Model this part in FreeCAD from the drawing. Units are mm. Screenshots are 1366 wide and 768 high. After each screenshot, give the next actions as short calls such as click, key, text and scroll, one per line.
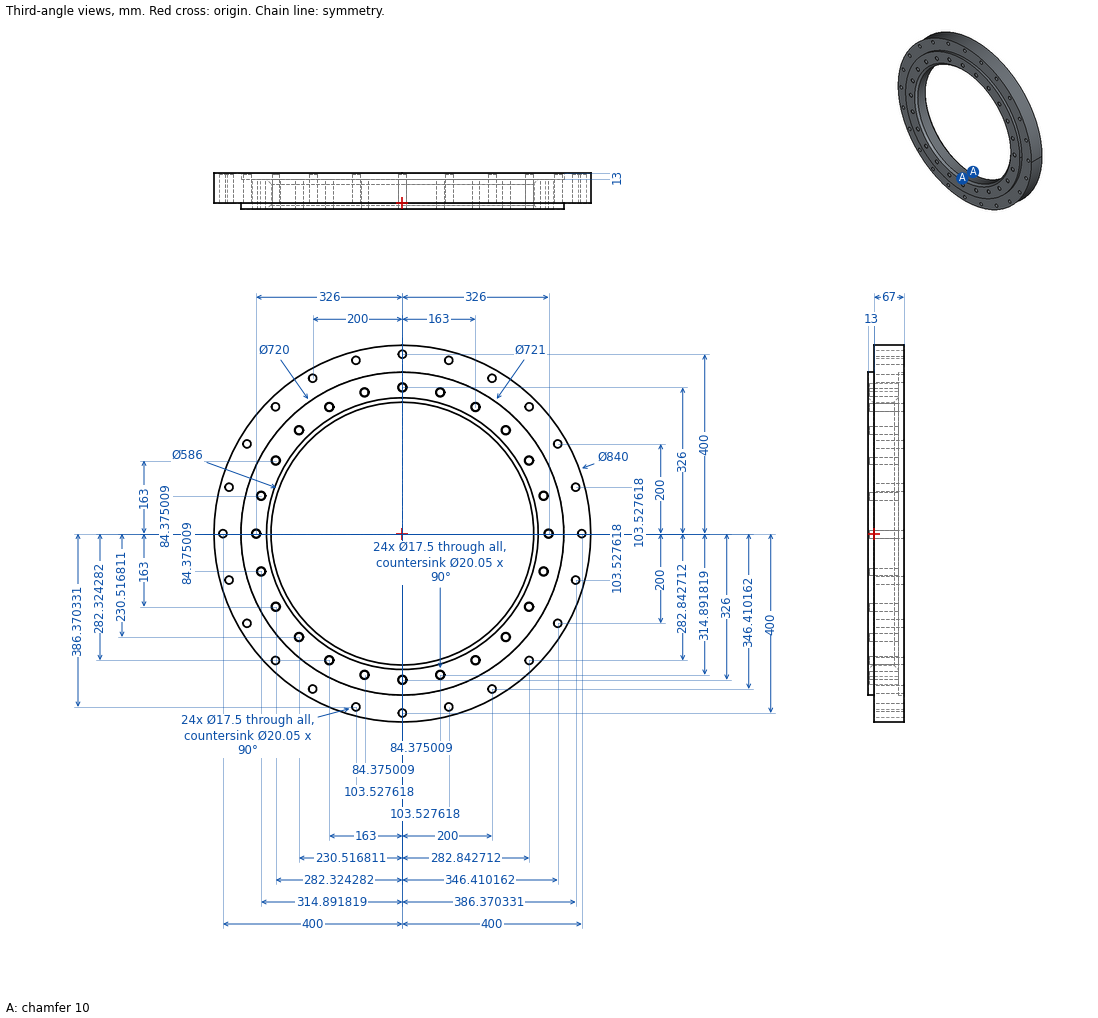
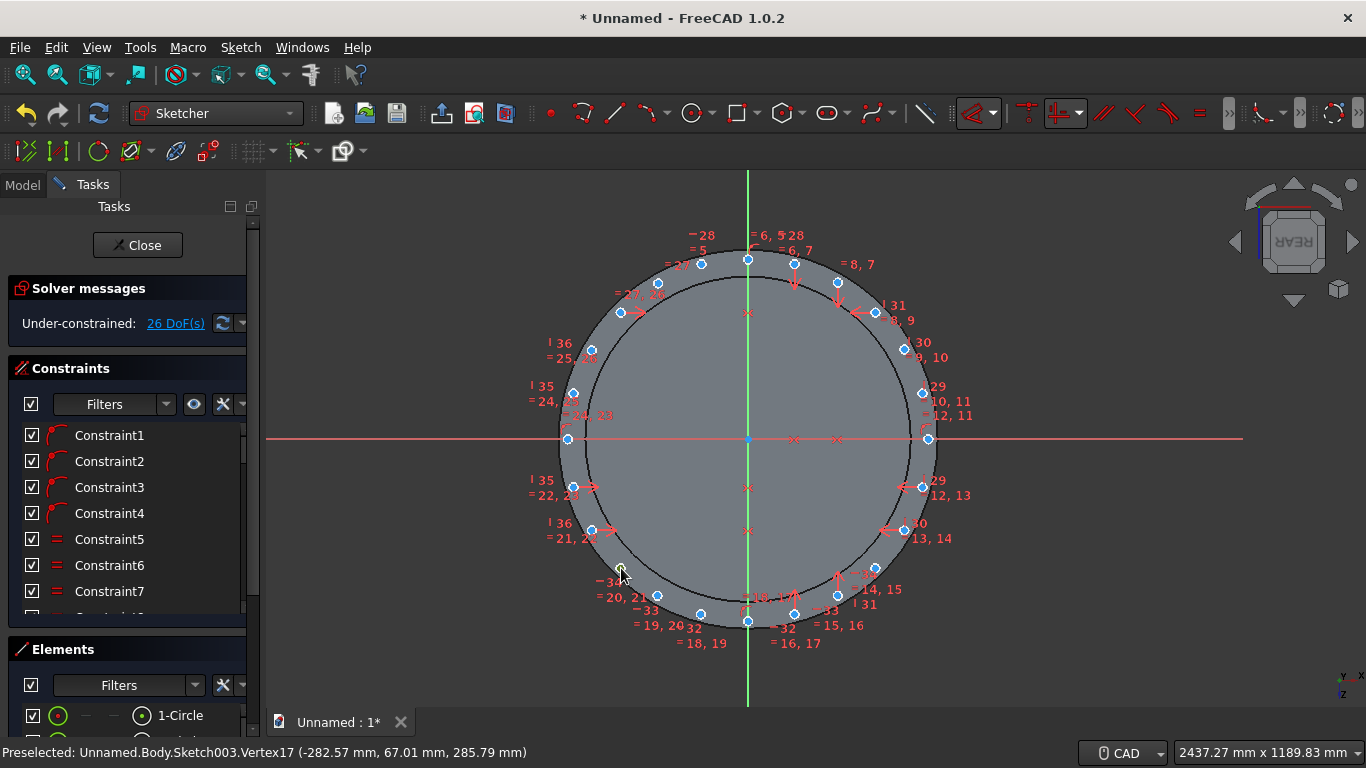
click(621, 313)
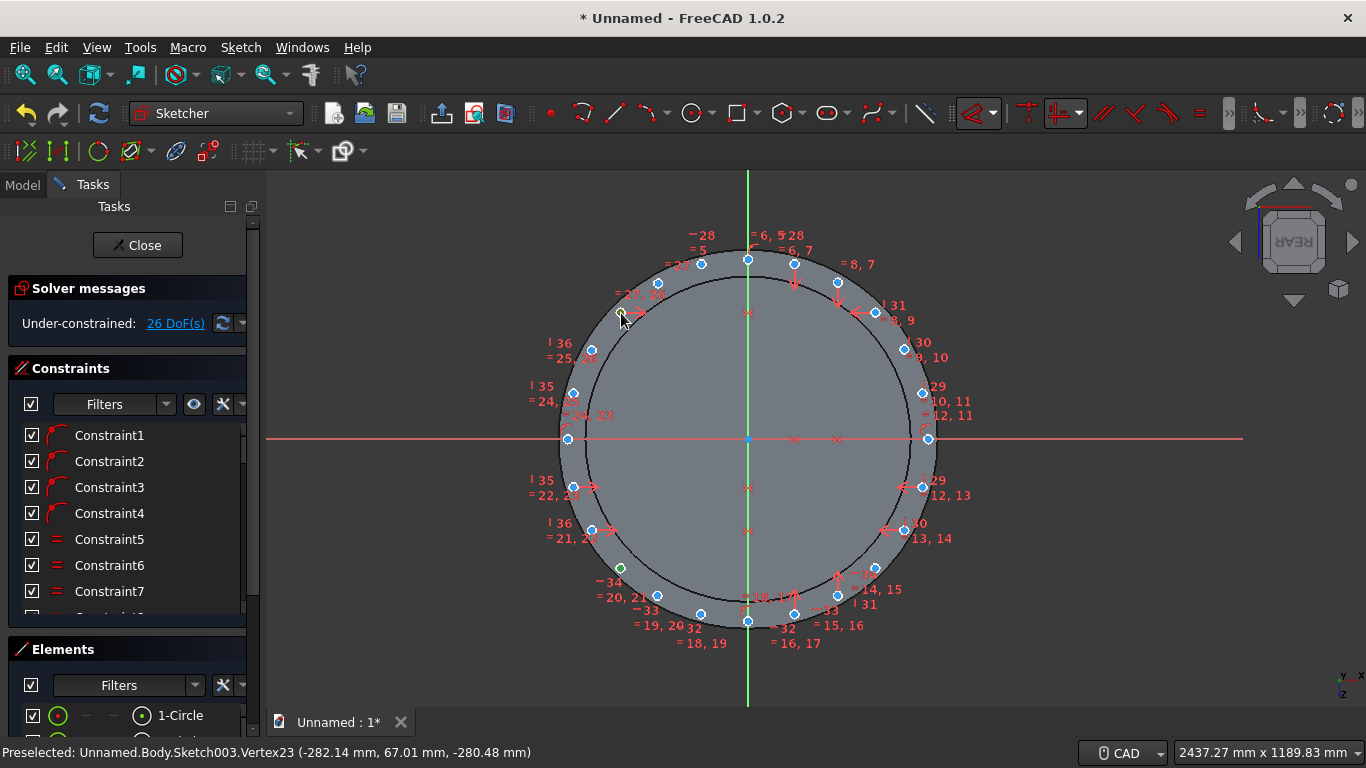
click(359, 439)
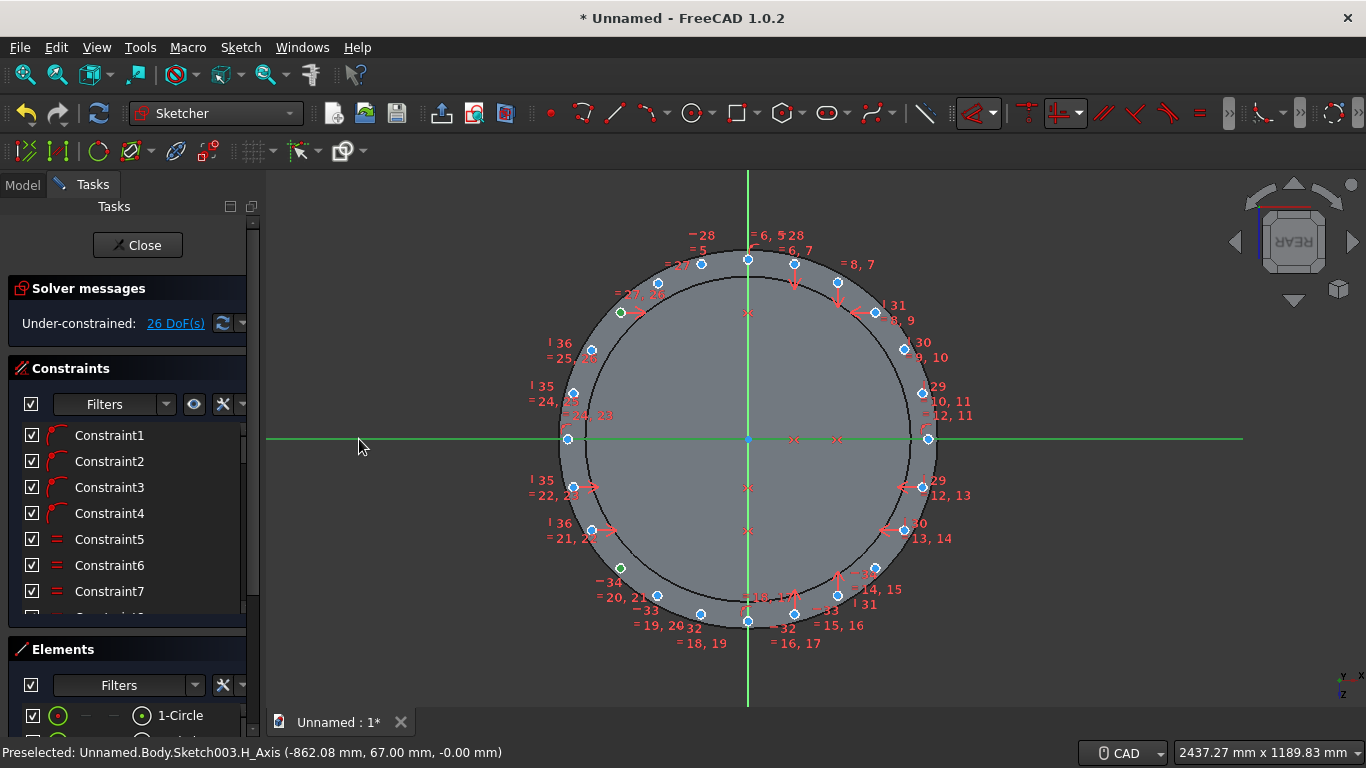
key(s)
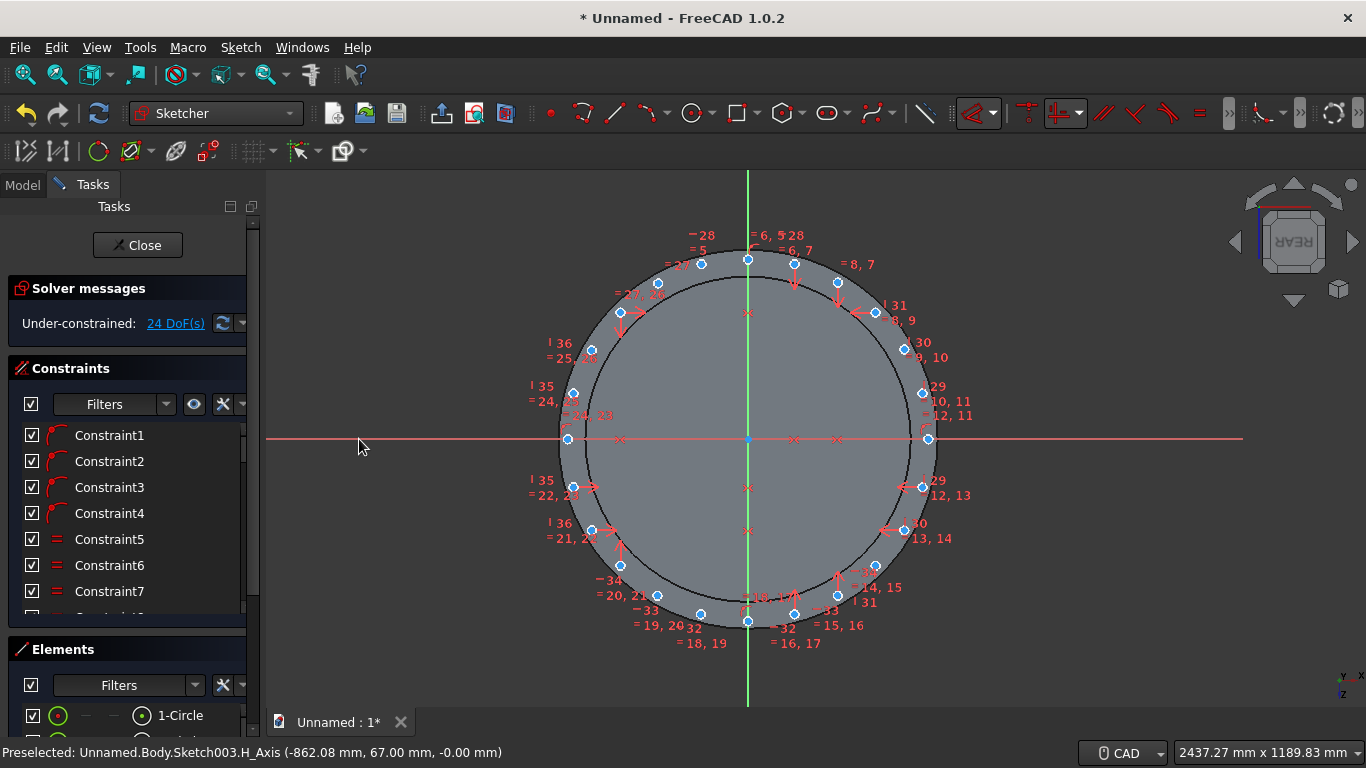
click(838, 283)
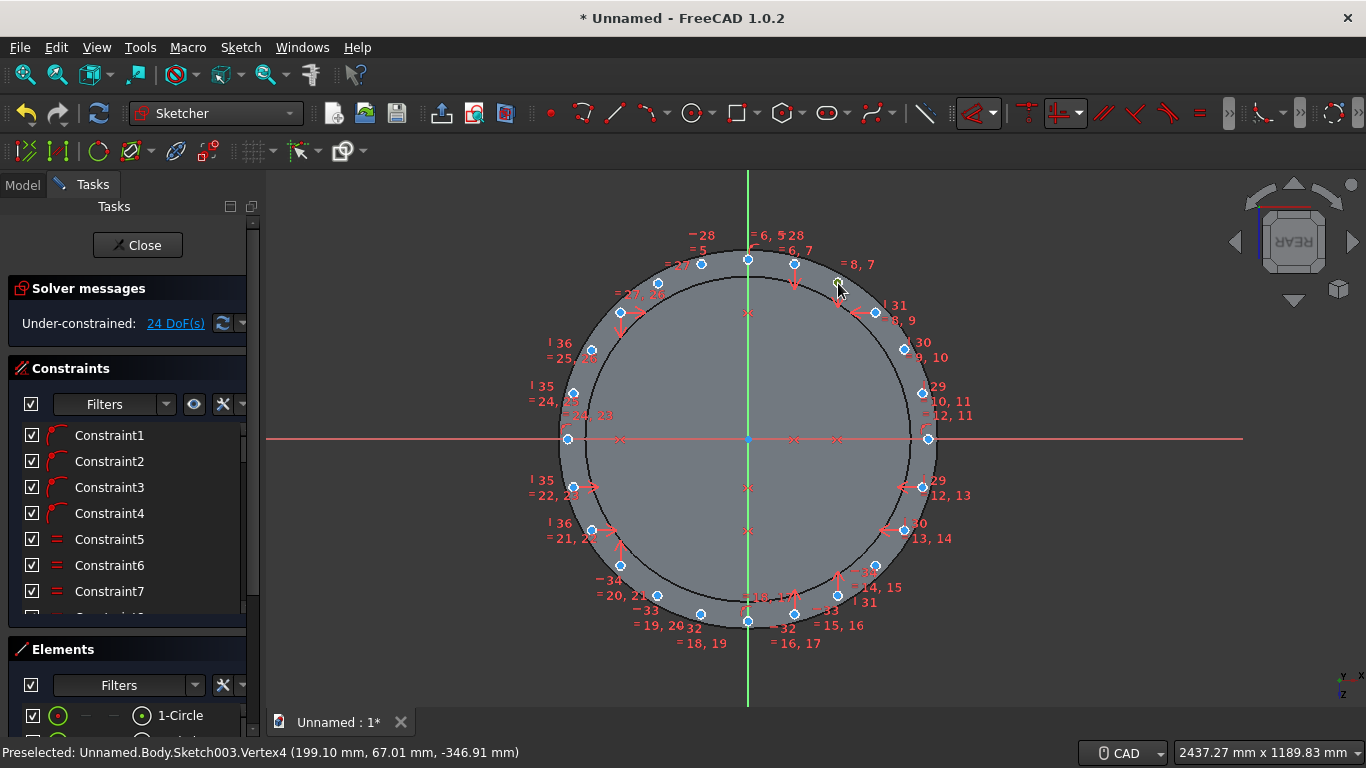
click(658, 283)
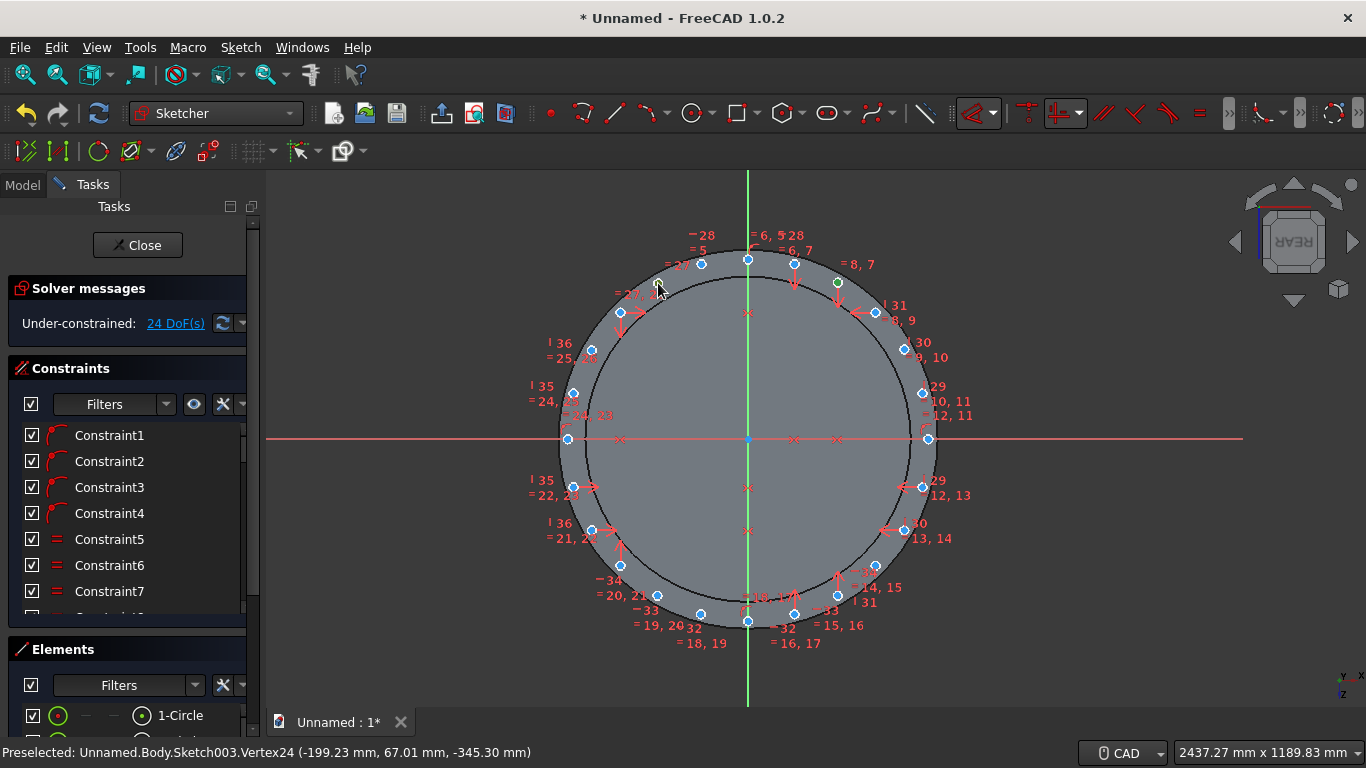
click(748, 576)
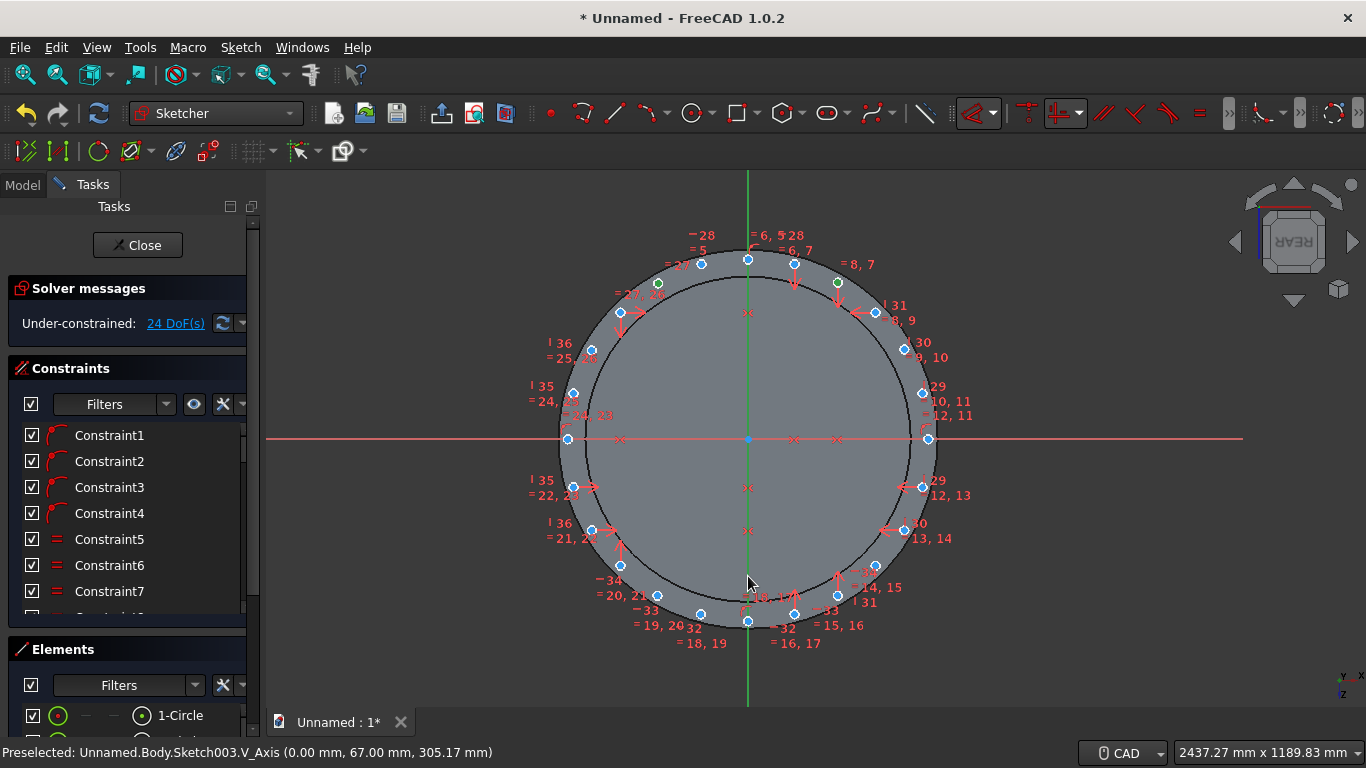
key(s)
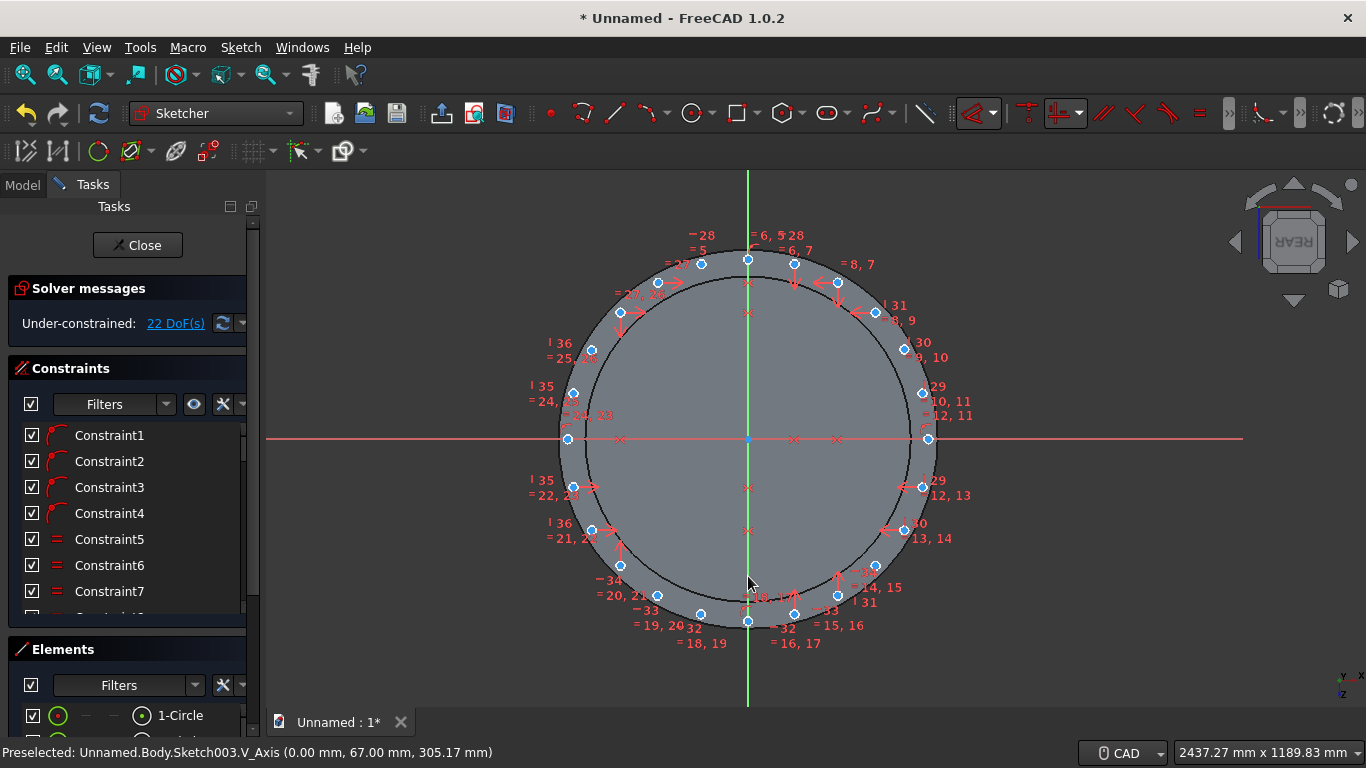
scroll(705, 261, up, 9)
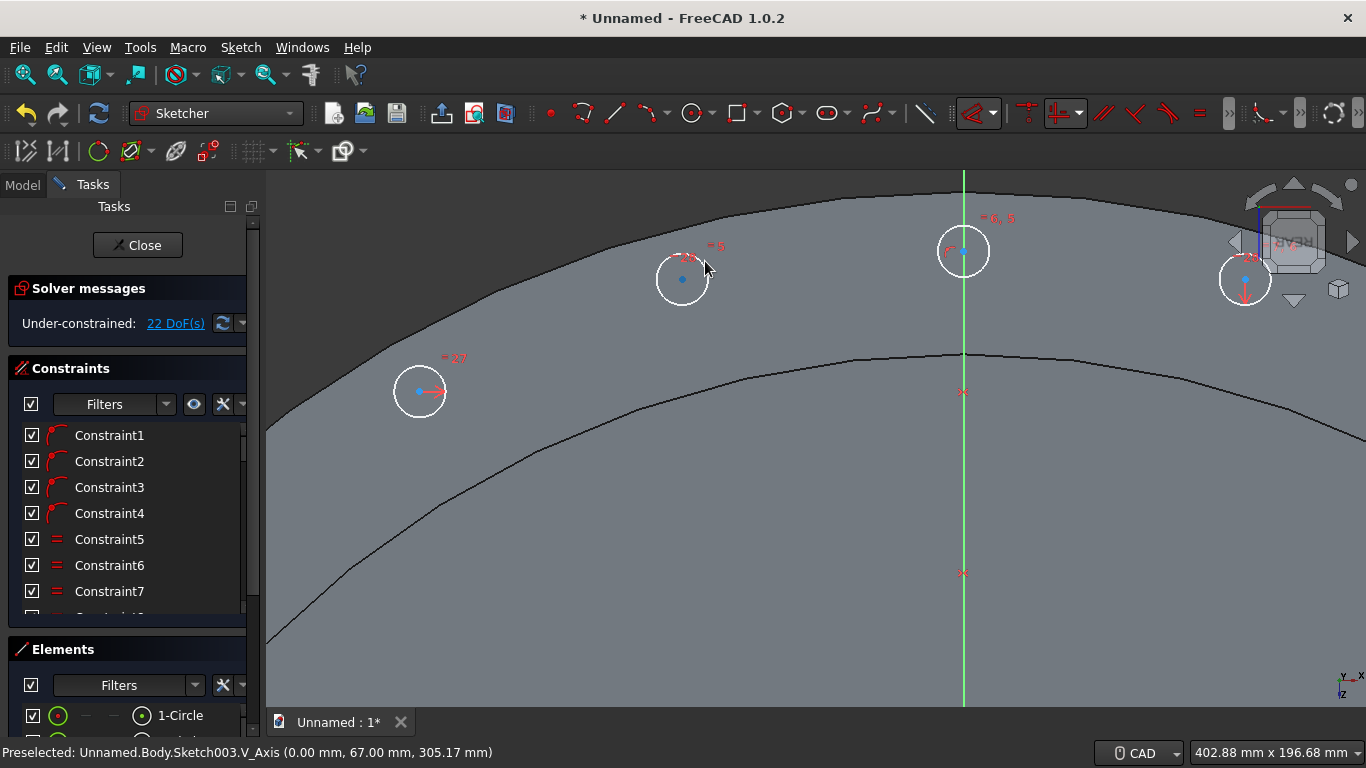
click(700, 261)